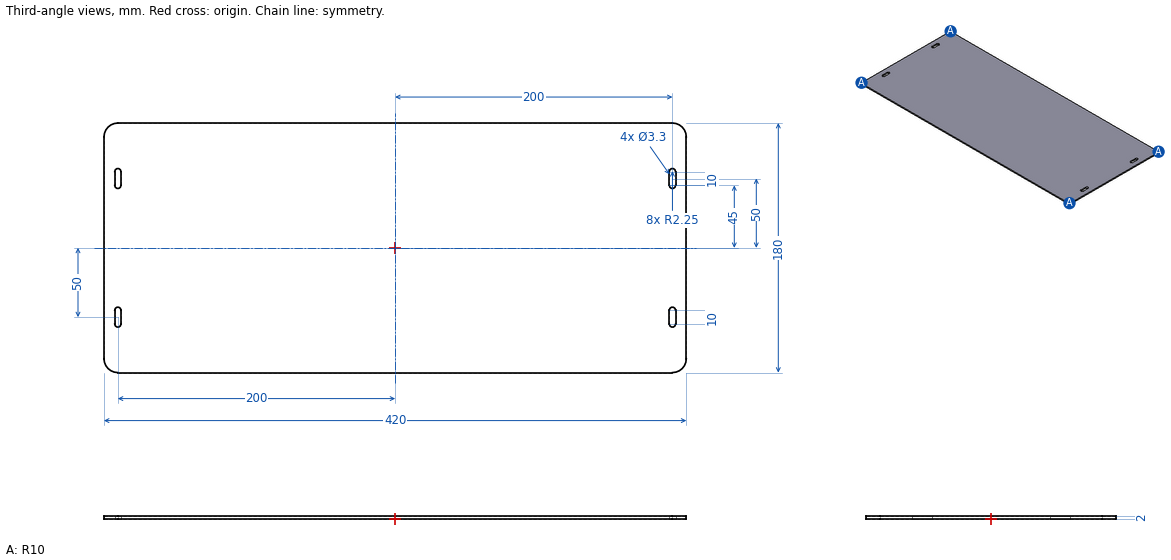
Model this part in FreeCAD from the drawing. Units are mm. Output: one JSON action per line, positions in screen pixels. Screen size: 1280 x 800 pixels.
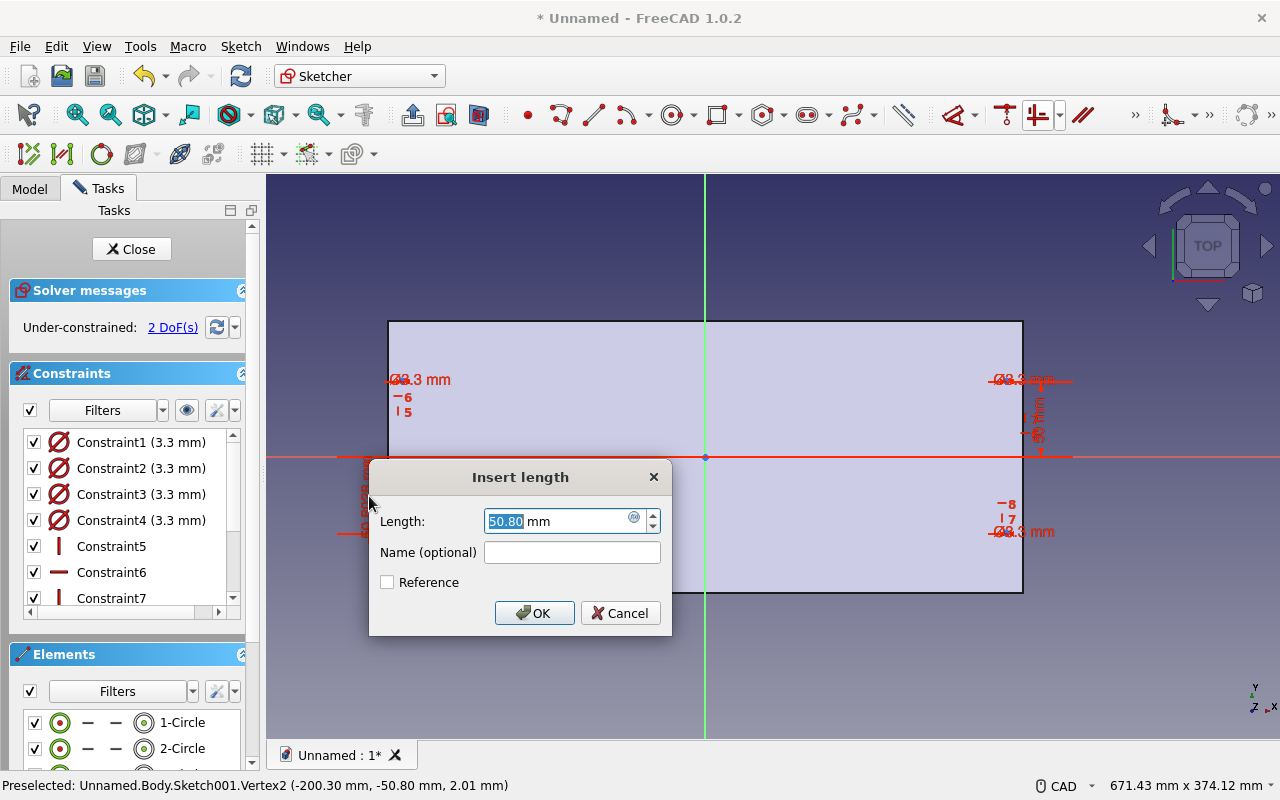
{"action": "type", "text": "50"}
{"action": "key", "text": "Return"}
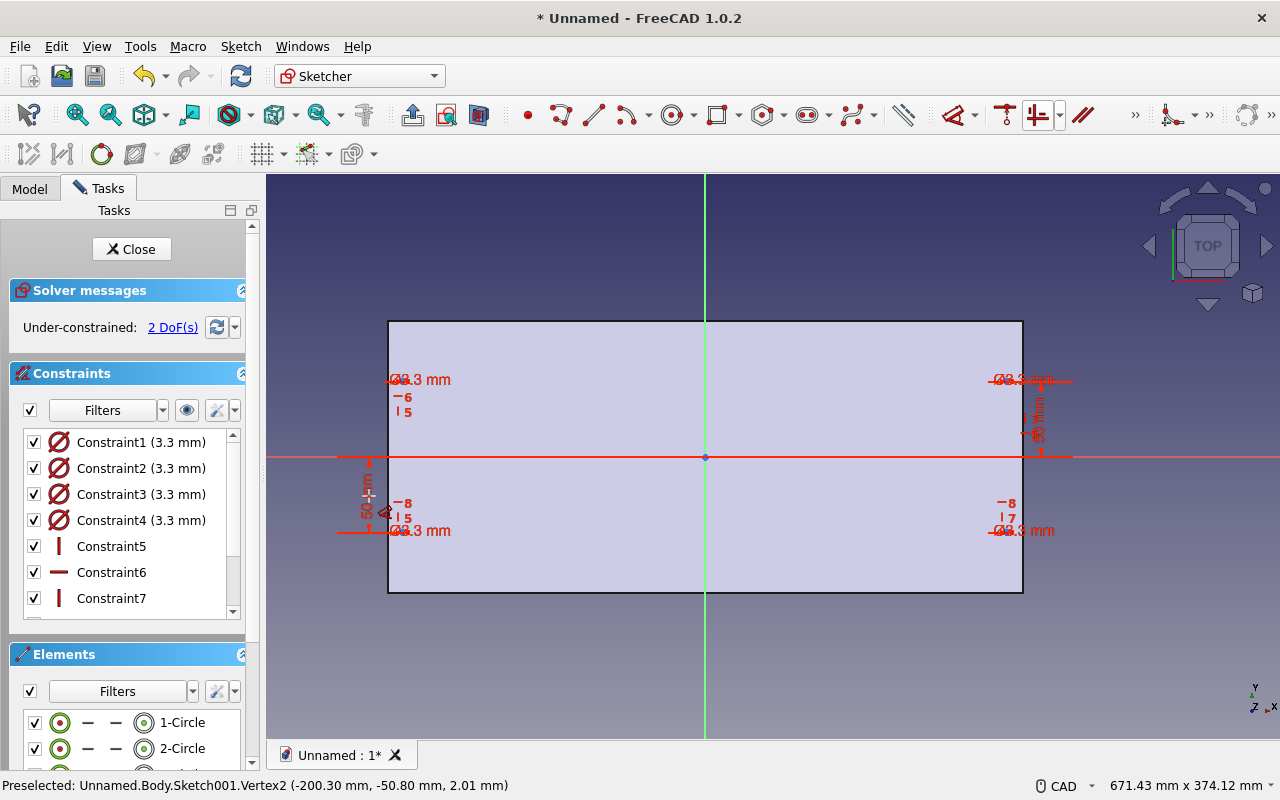
{"action": "left_click", "coordinate": [1007, 382]}
{"action": "left_click", "coordinate": [856, 348]}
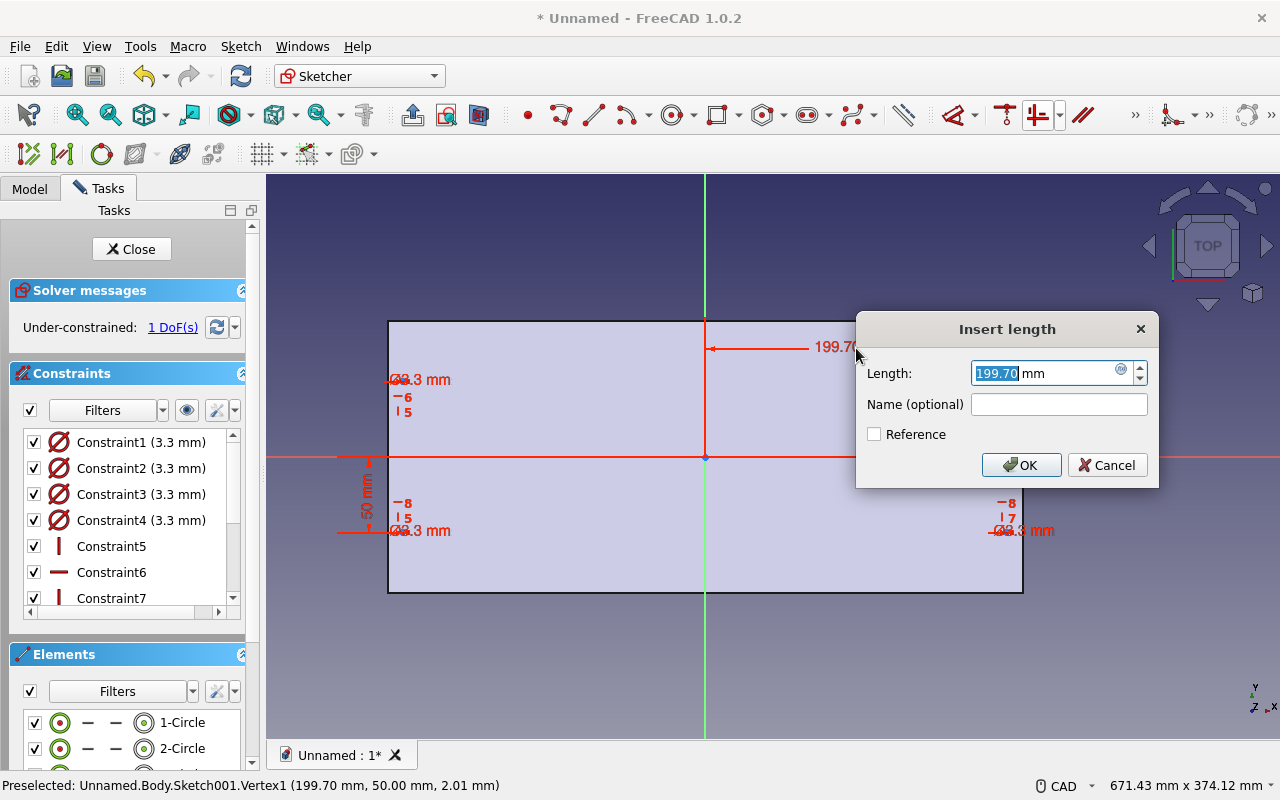
{"action": "type", "text": "200"}
{"action": "key", "text": "Return"}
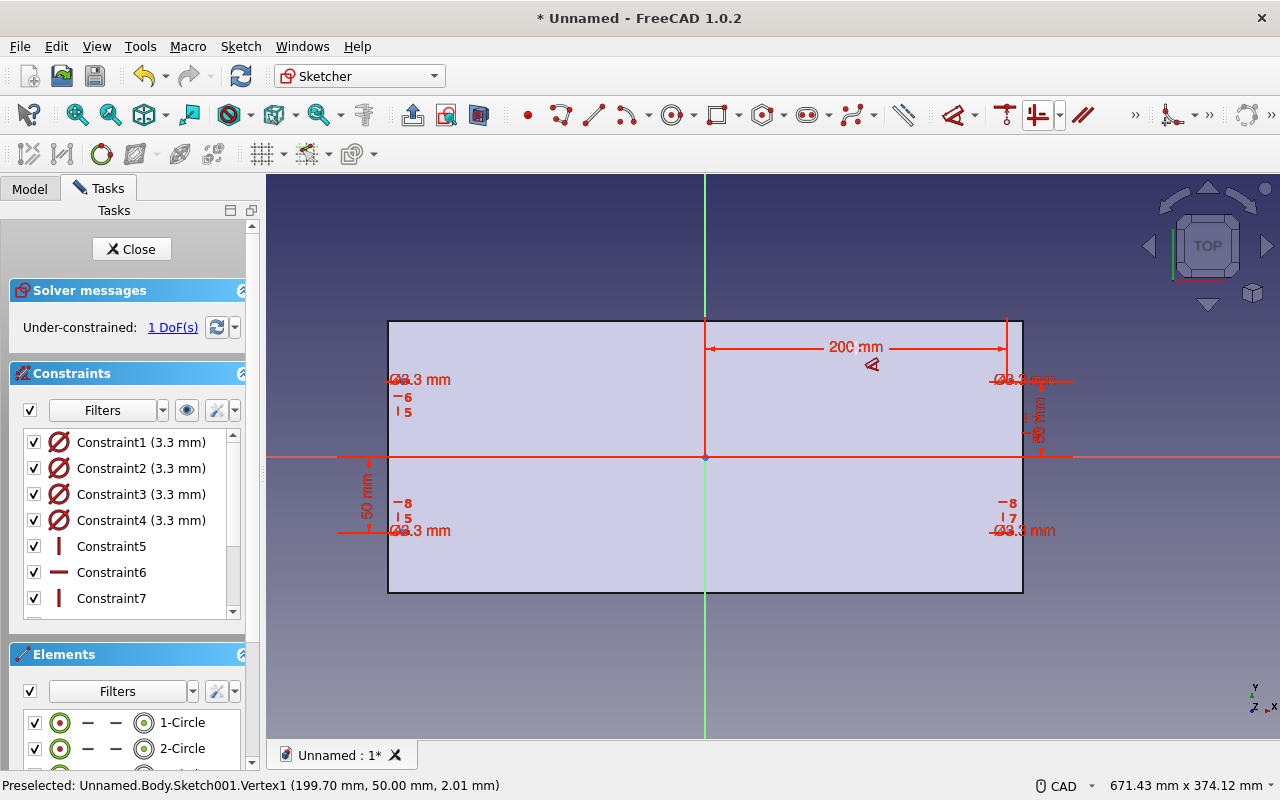
{"action": "left_click", "coordinate": [403, 533]}
{"action": "left_click", "coordinate": [554, 567]}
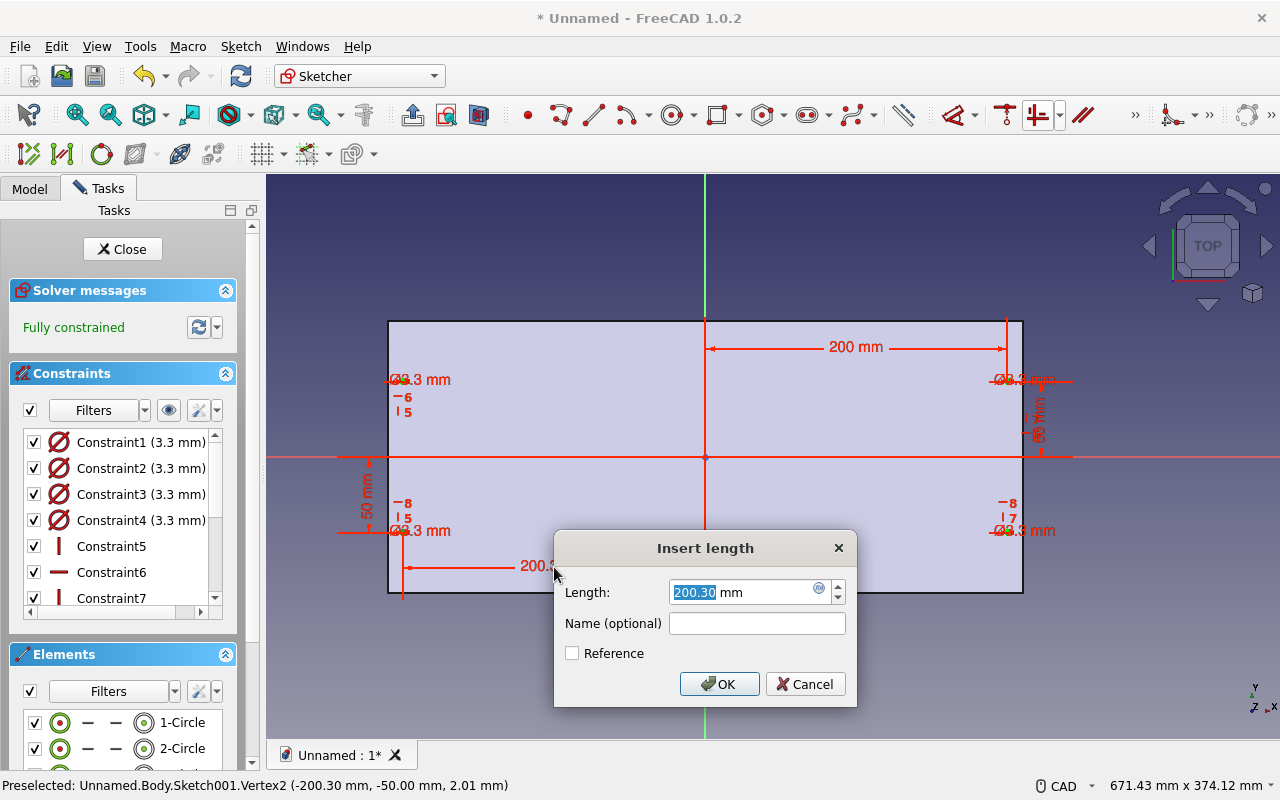
{"action": "type", "text": "200"}
{"action": "key", "text": "Return"}
{"action": "key", "text": "Escape"}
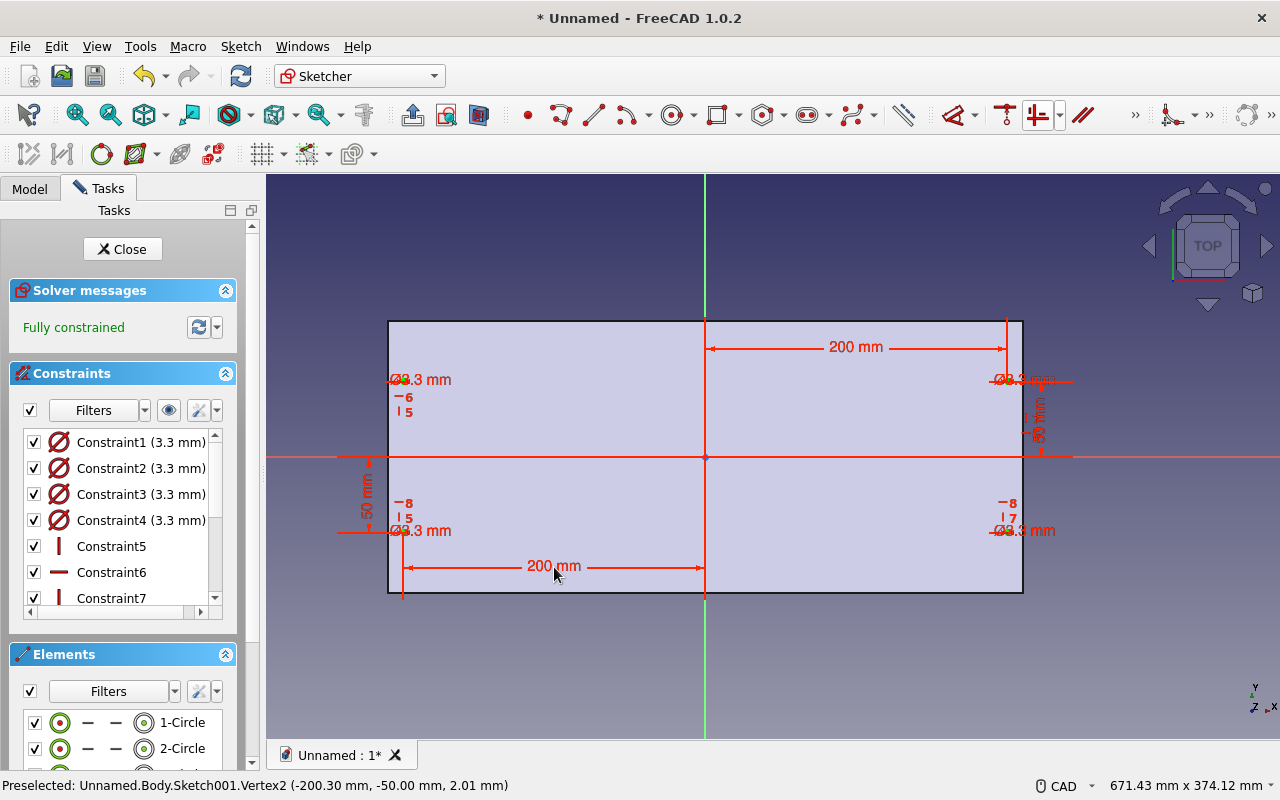
{"action": "left_click", "coordinate": [123, 249]}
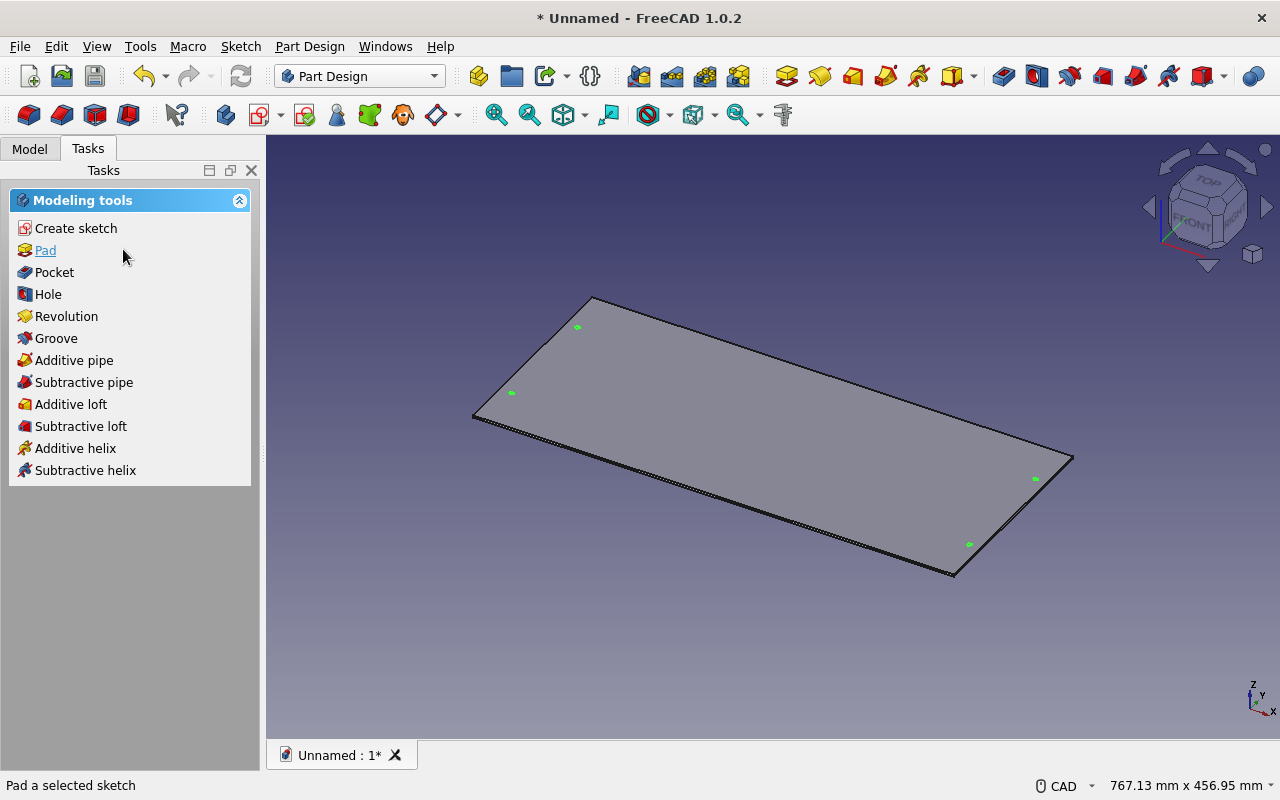
{"action": "left_click", "coordinate": [1004, 76]}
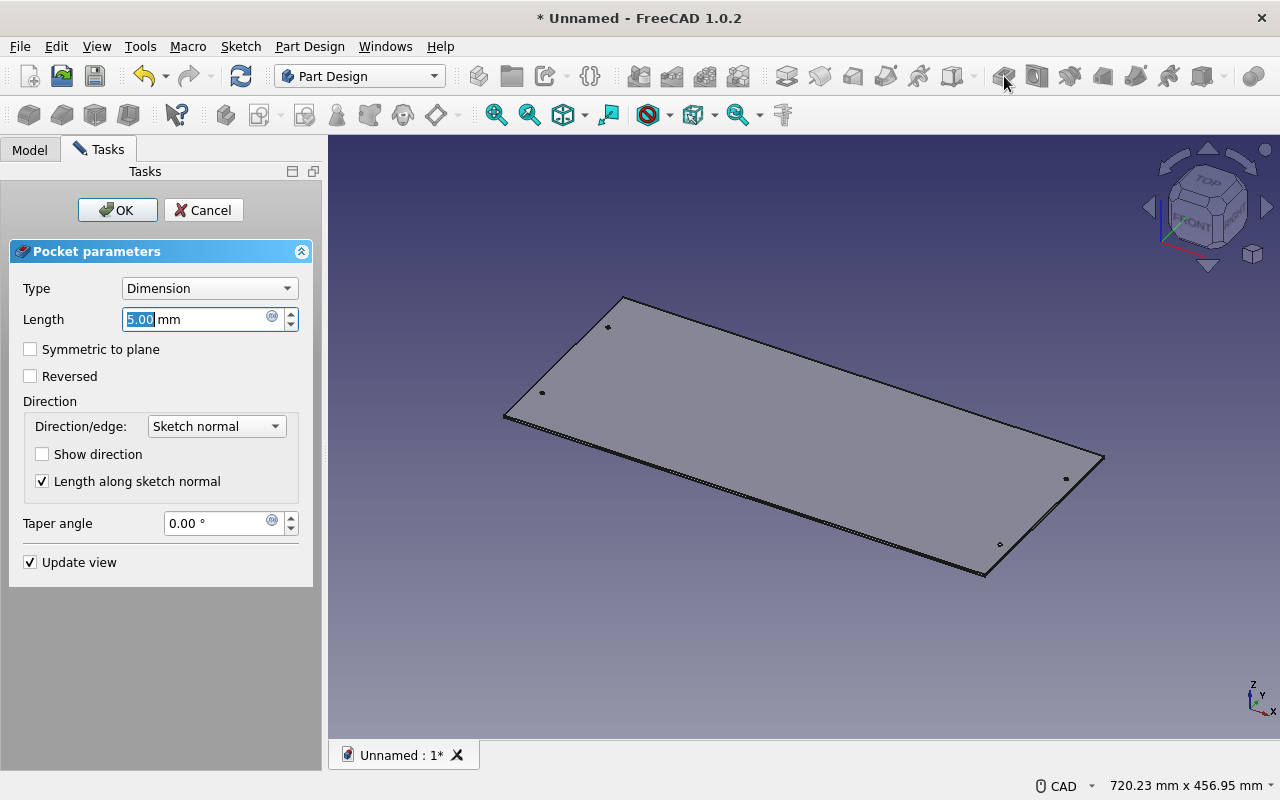
{"action": "left_click", "coordinate": [210, 288]}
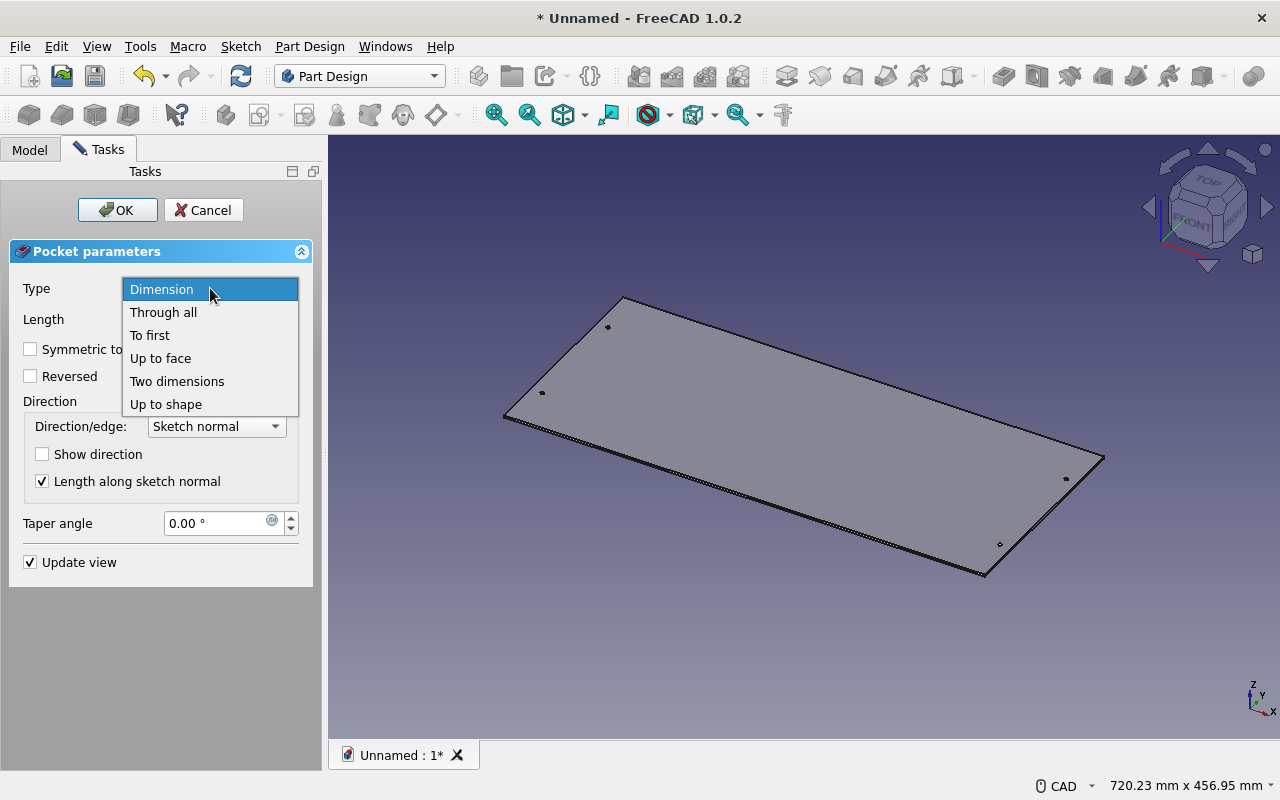
{"action": "left_click", "coordinate": [208, 312]}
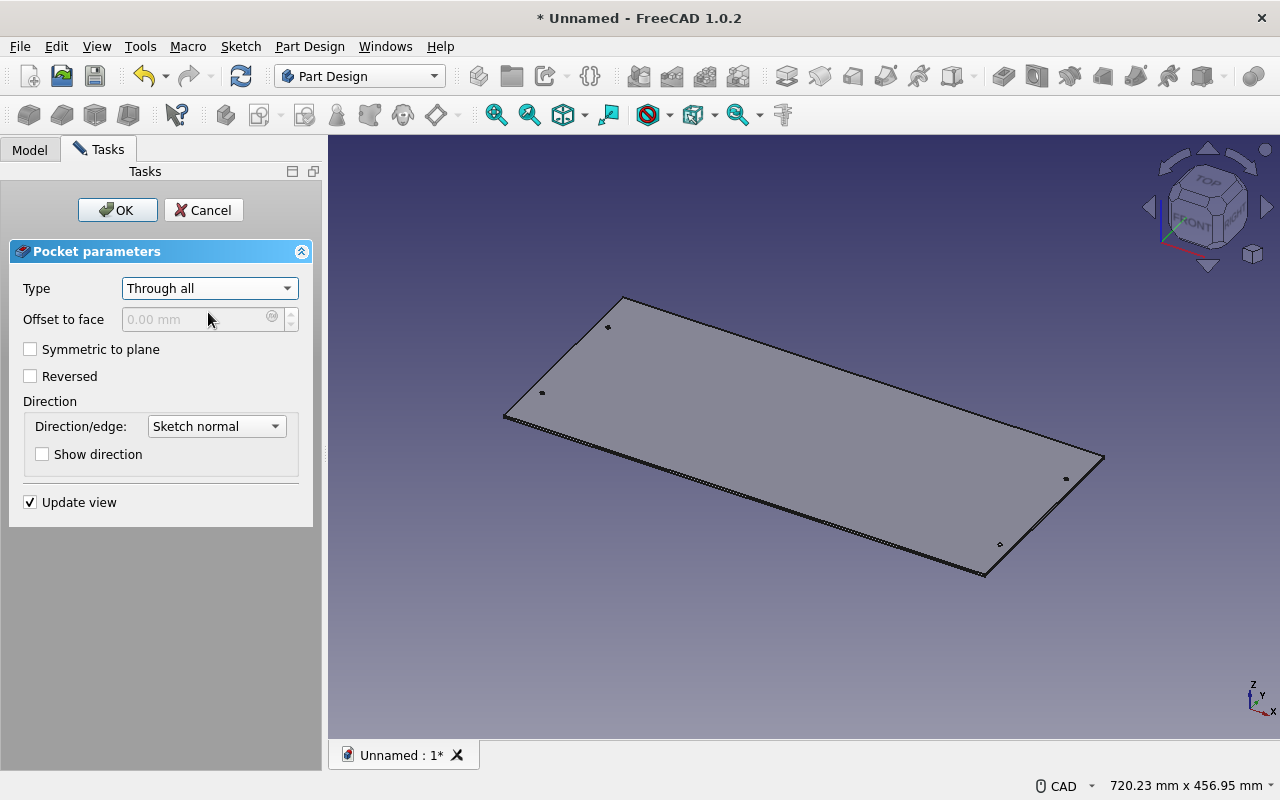
{"action": "left_click", "coordinate": [118, 210]}